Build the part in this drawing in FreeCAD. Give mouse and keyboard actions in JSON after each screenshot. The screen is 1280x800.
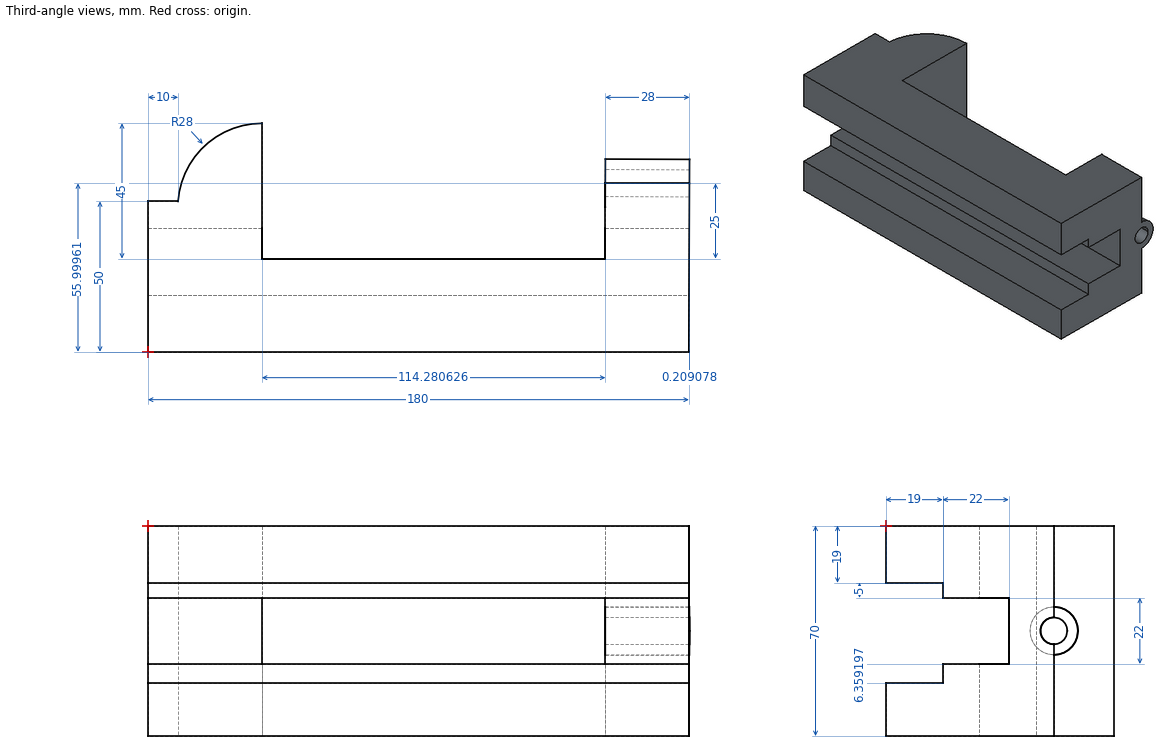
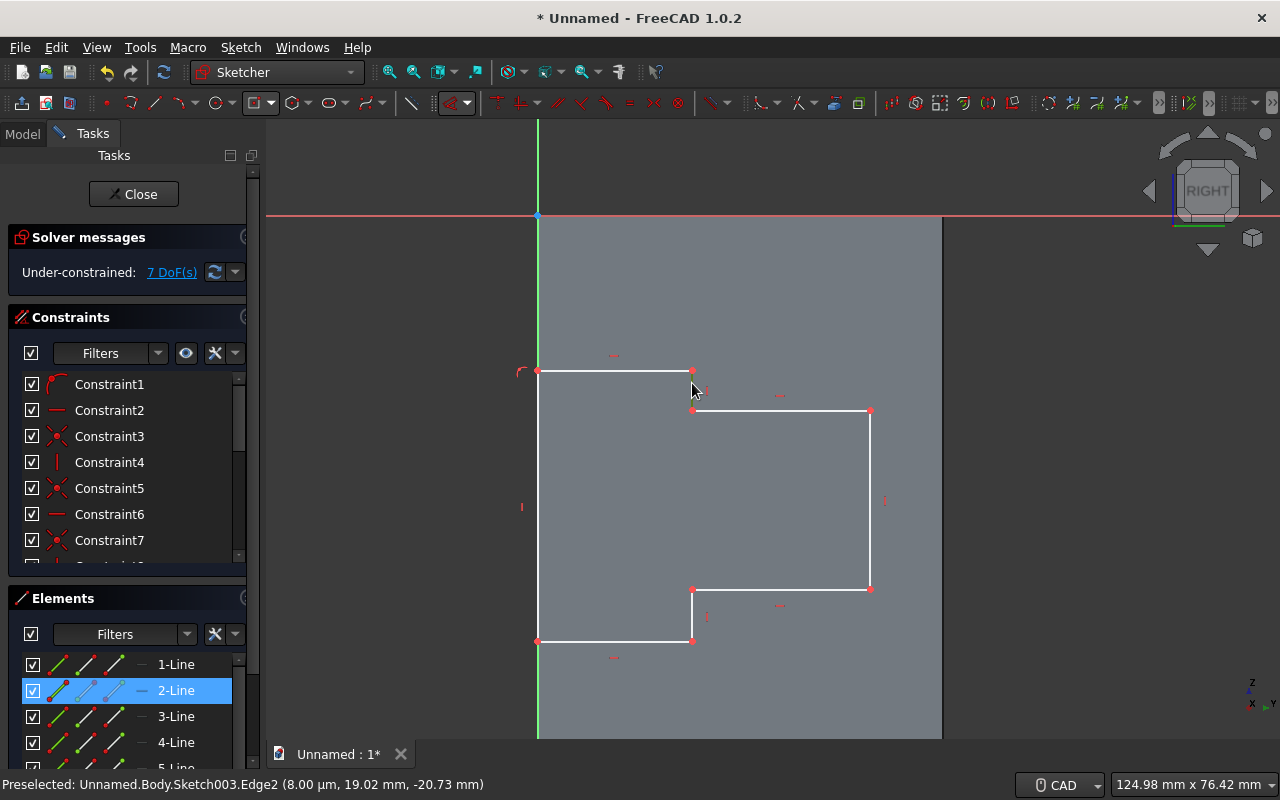
{"action": "key", "text": "i"}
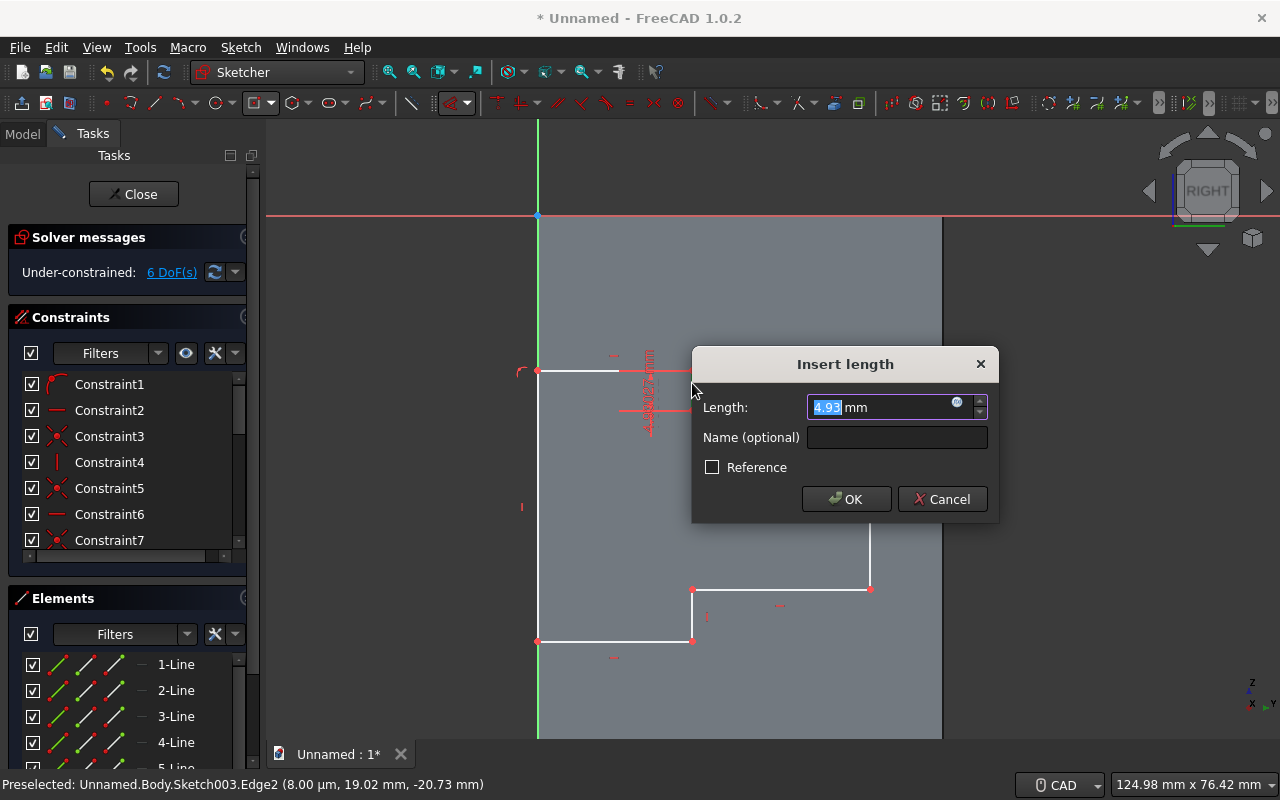
{"action": "type", "text": "5"}
{"action": "key", "text": "Return"}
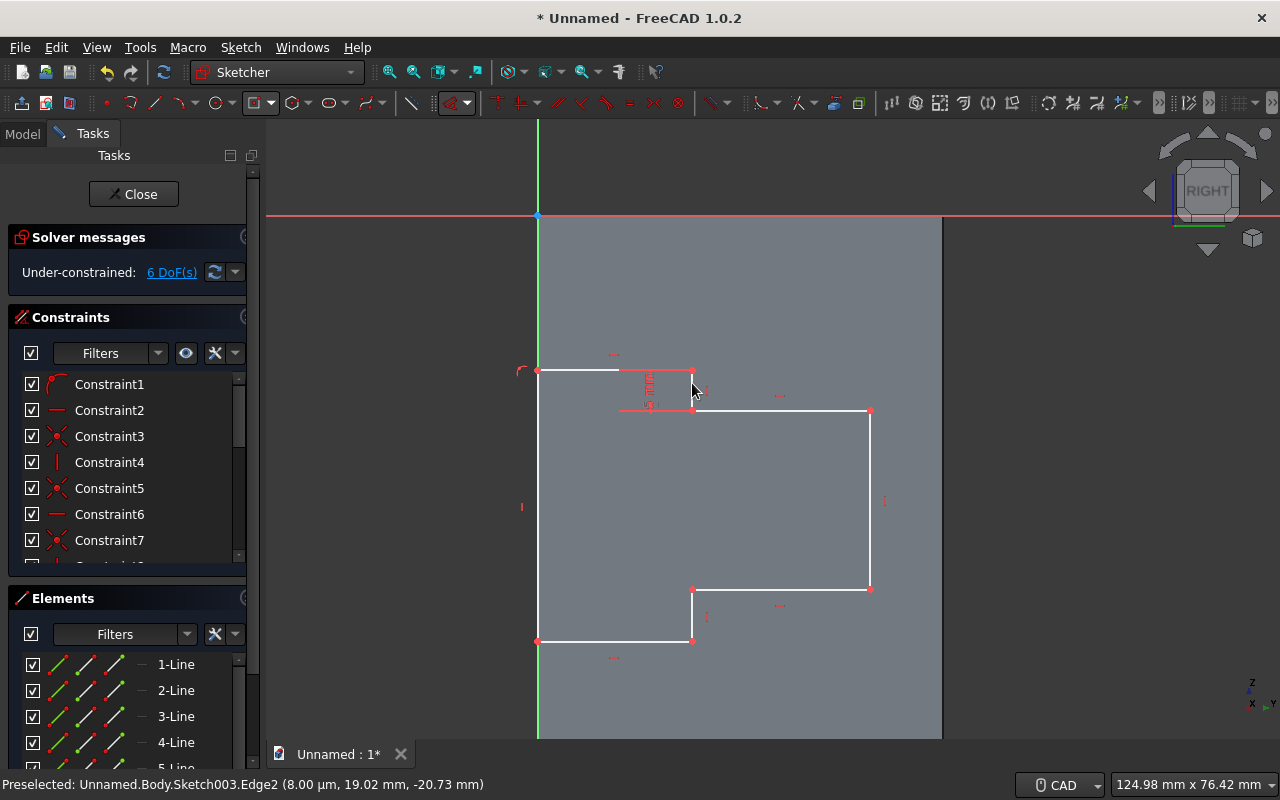
{"action": "left_click", "coordinate": [584, 370]}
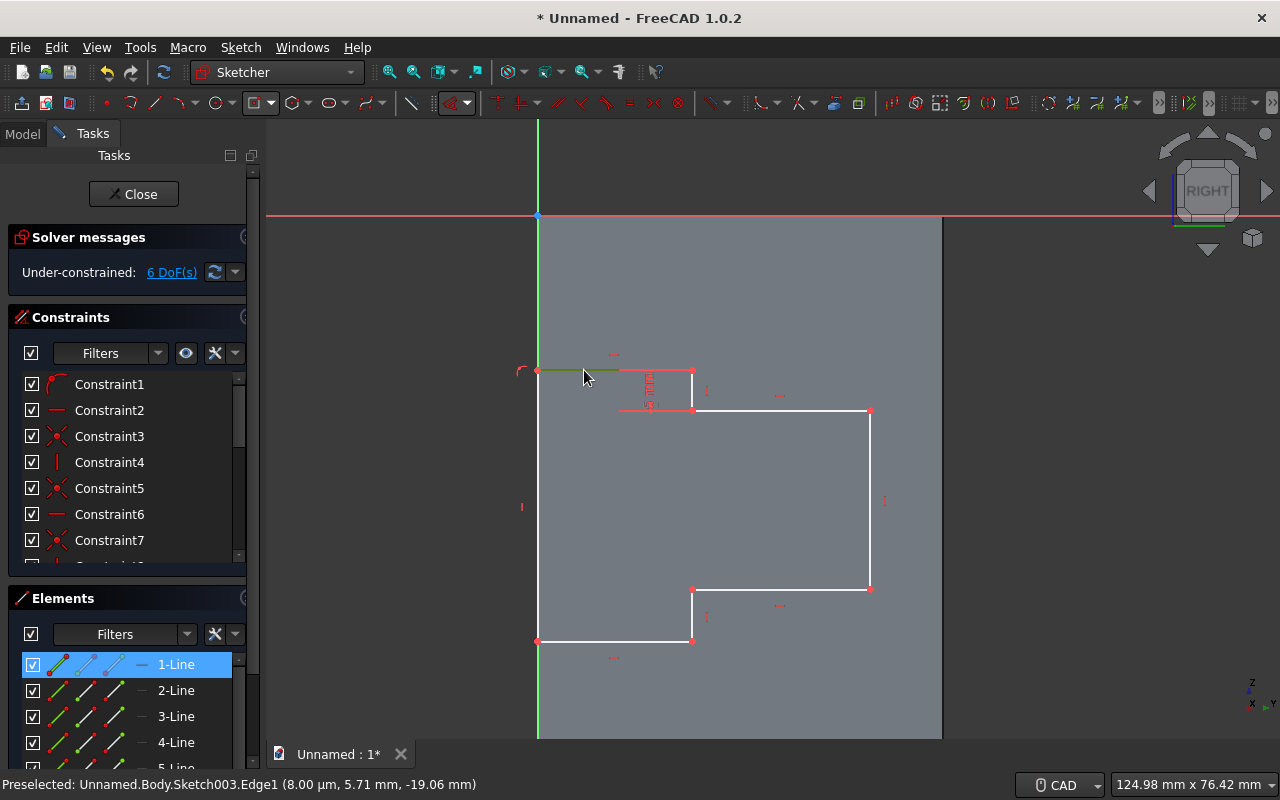
{"action": "left_click", "coordinate": [470, 104]}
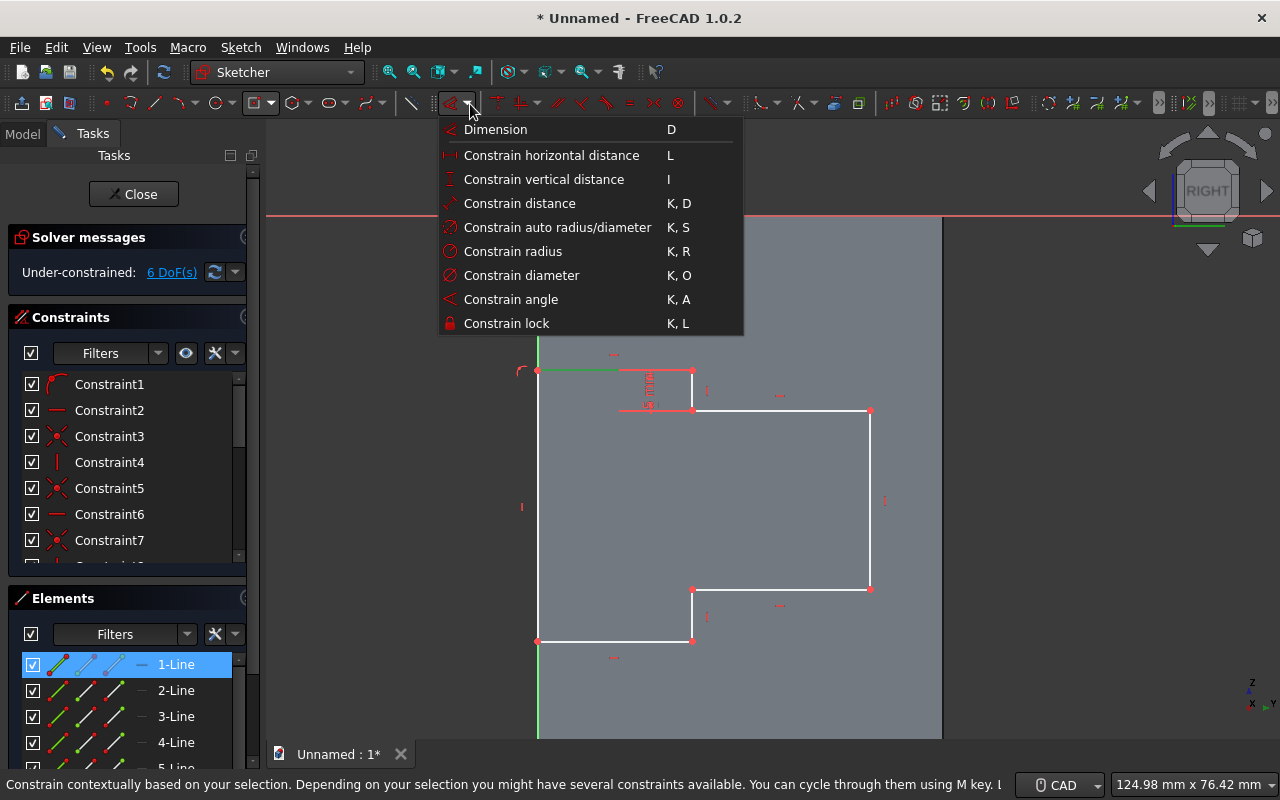
{"action": "left_click", "coordinate": [591, 155]}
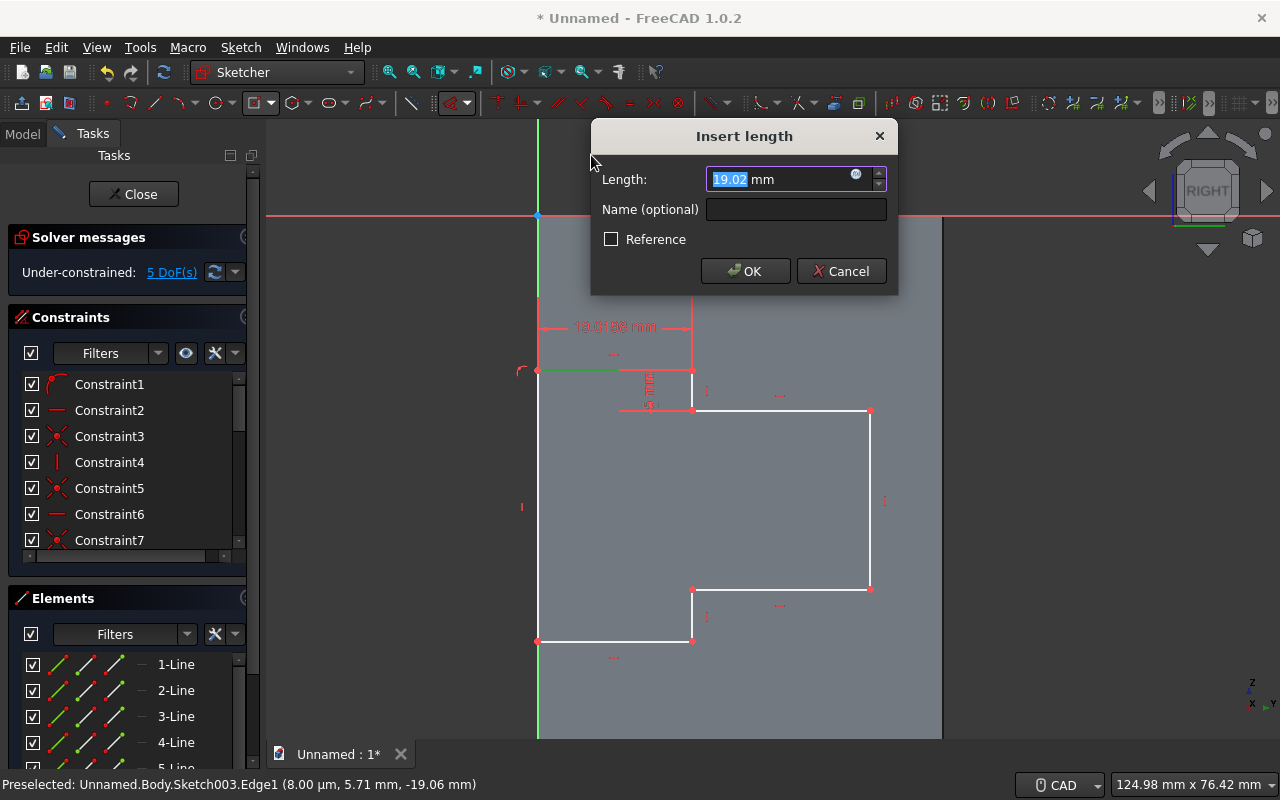
{"action": "type", "text": "19"}
{"action": "key", "text": "Return"}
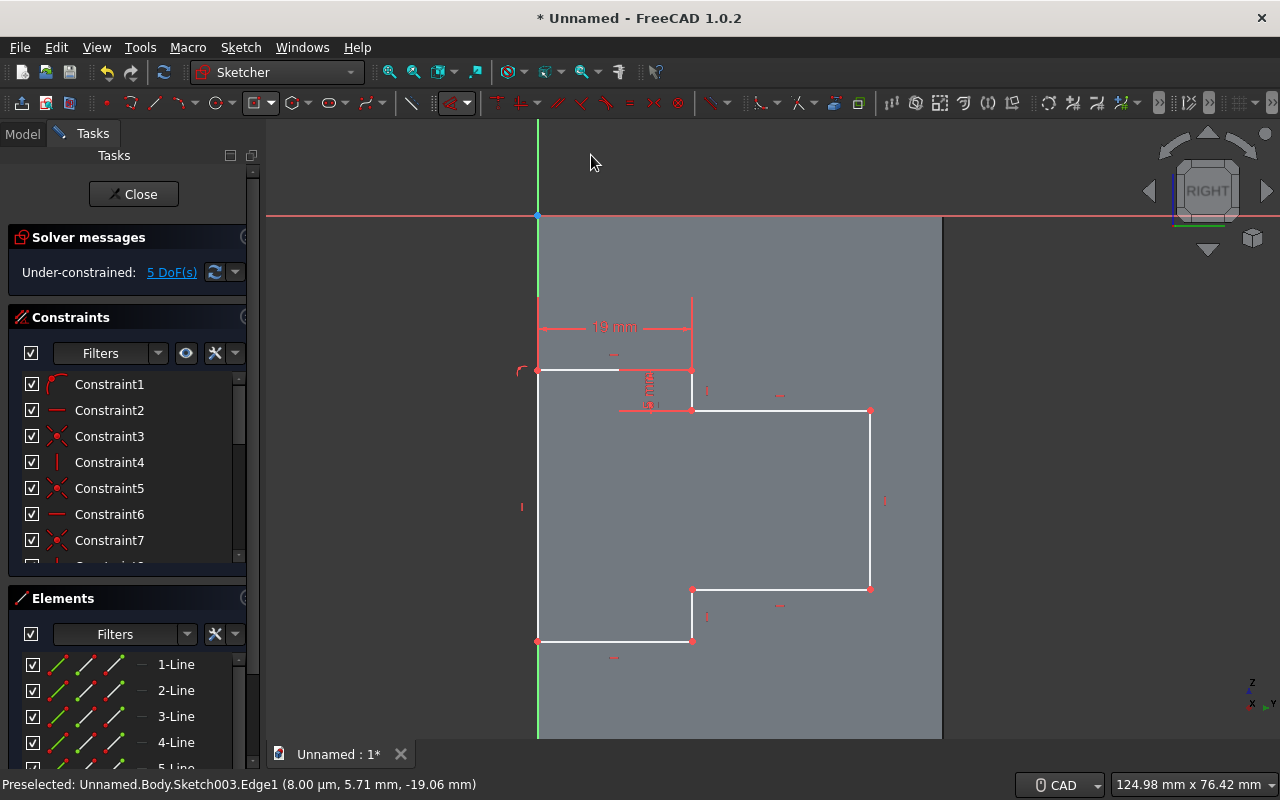
{"action": "left_click", "coordinate": [745, 411]}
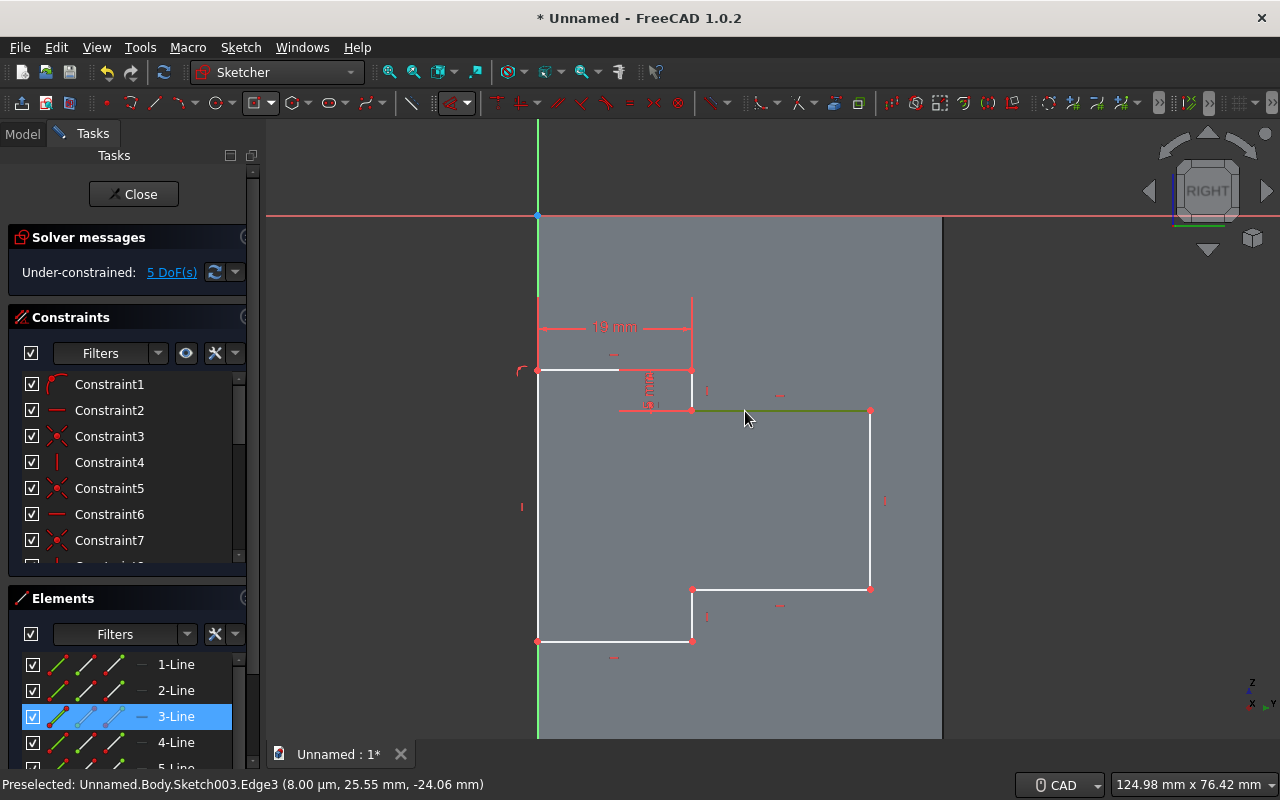
{"action": "key", "text": "l"}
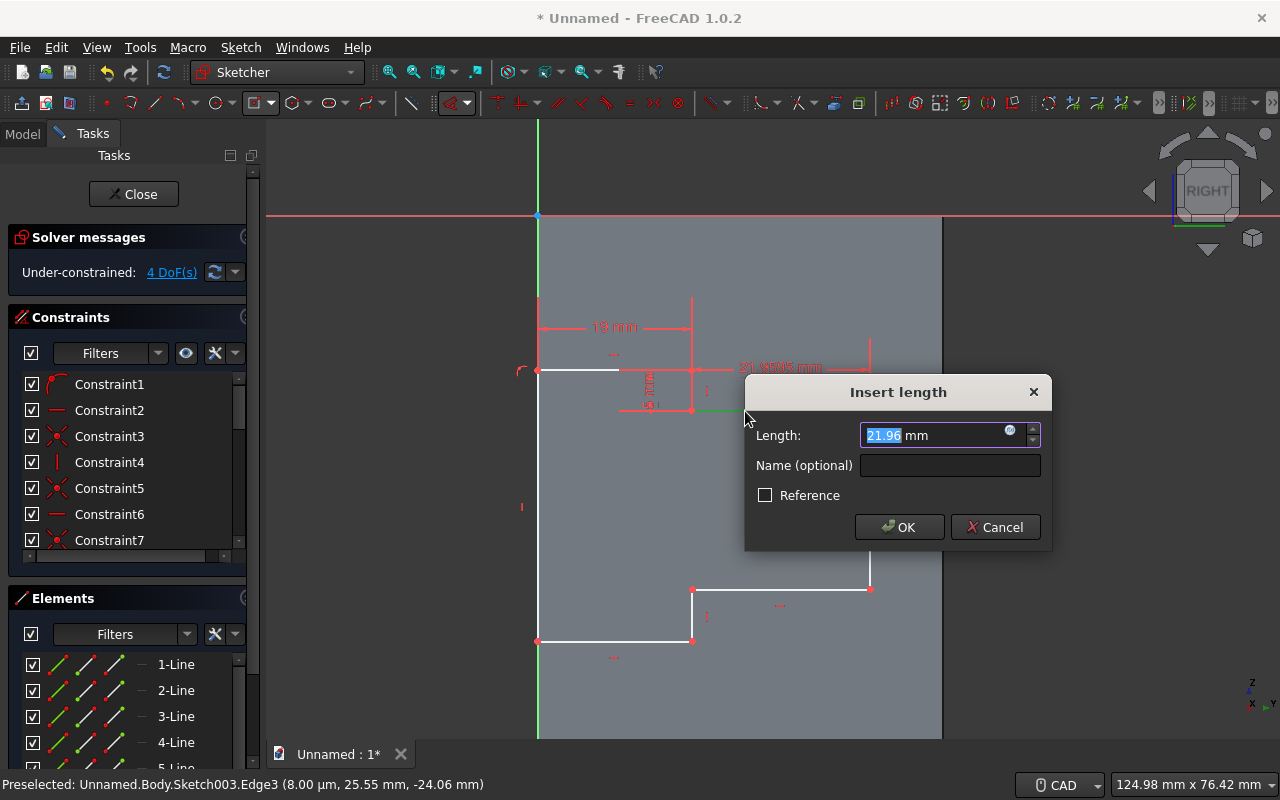
{"action": "type", "text": "22"}
{"action": "key", "text": "Return"}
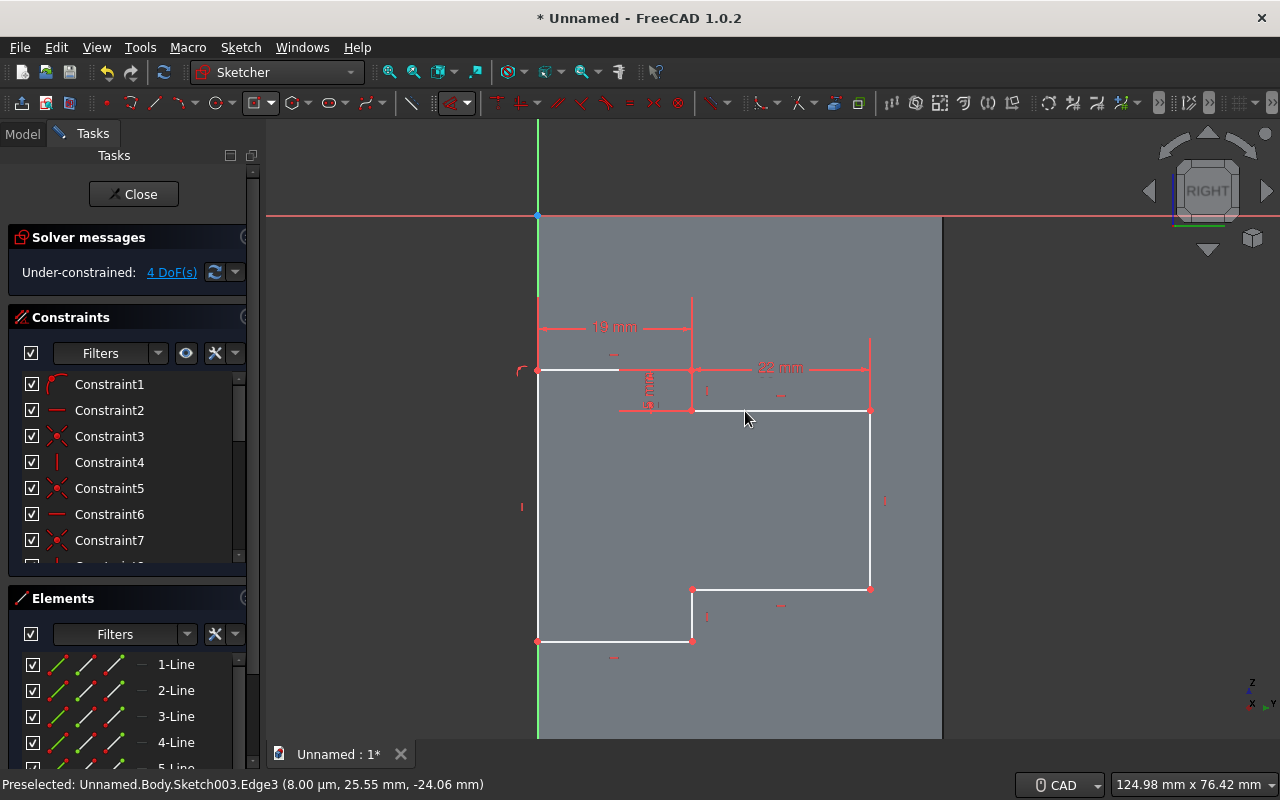
{"action": "left_click", "coordinate": [870, 465]}